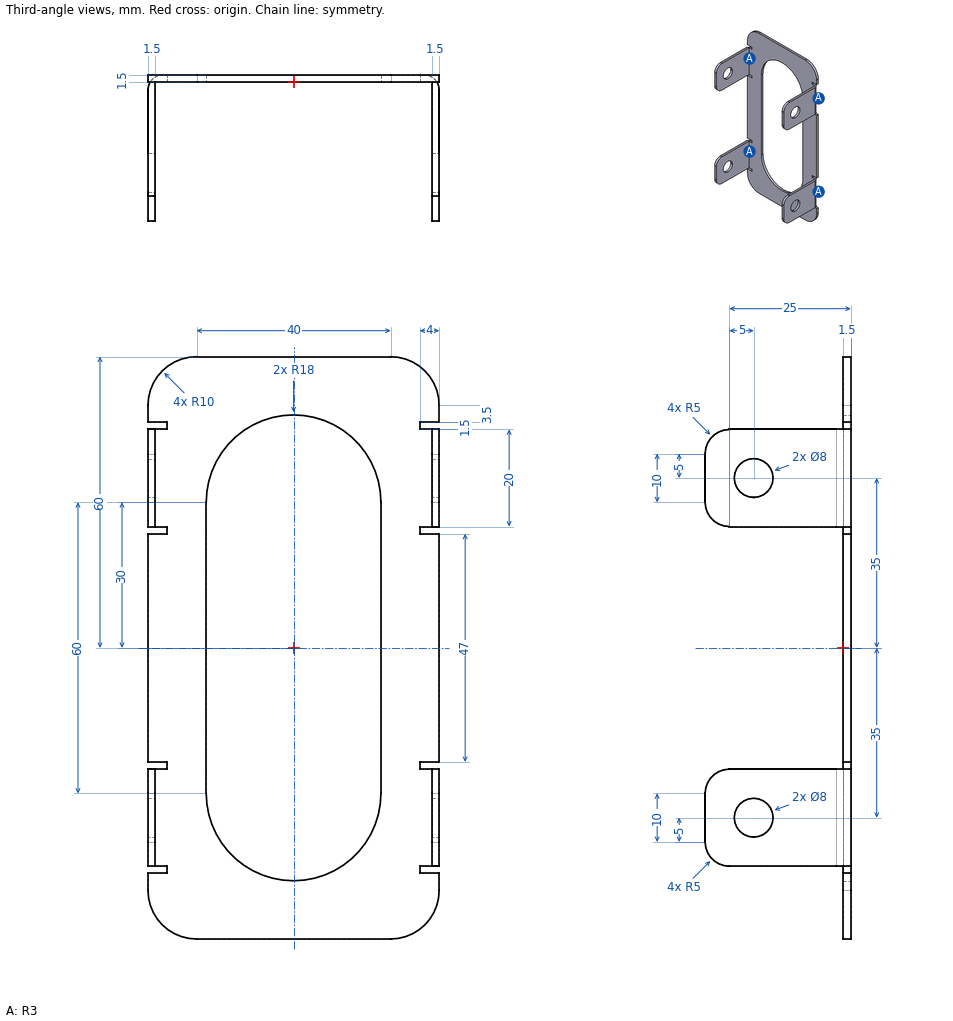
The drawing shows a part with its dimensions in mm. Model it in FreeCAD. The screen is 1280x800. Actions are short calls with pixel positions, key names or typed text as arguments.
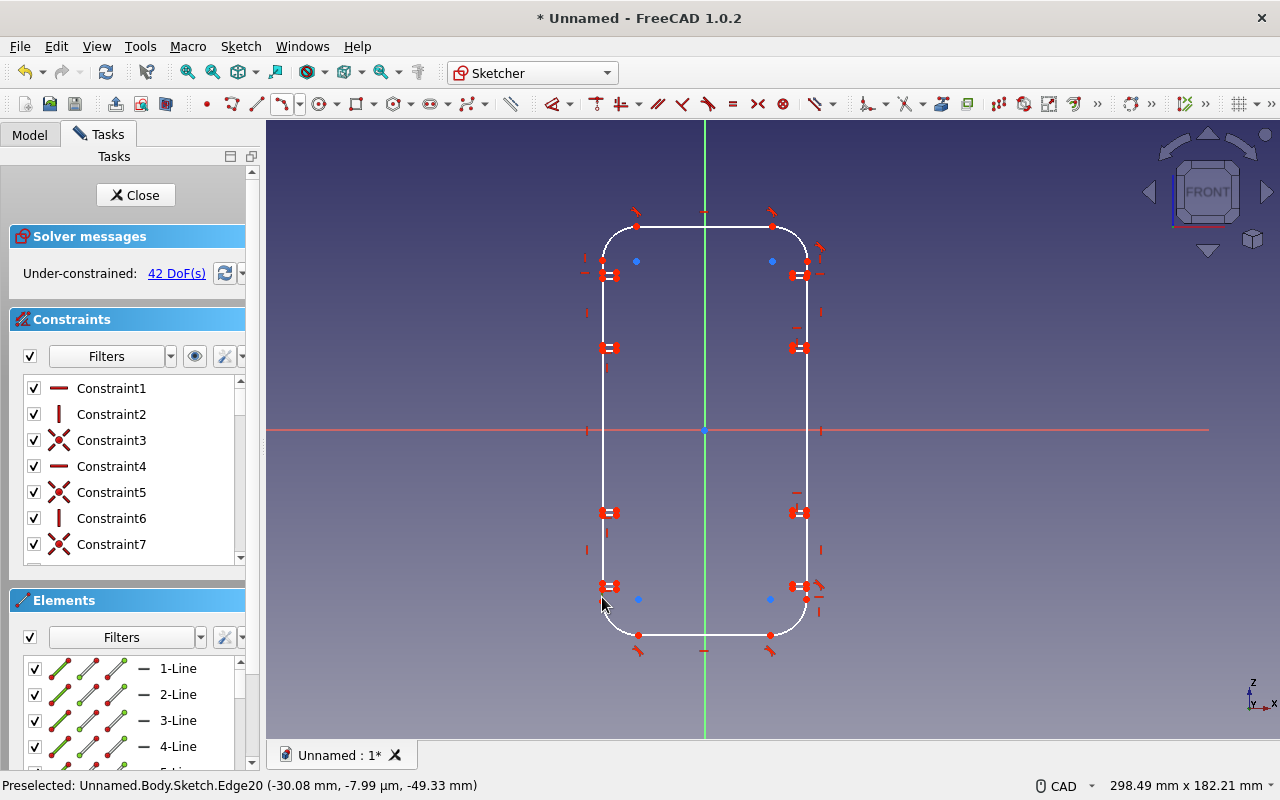
click(607, 617)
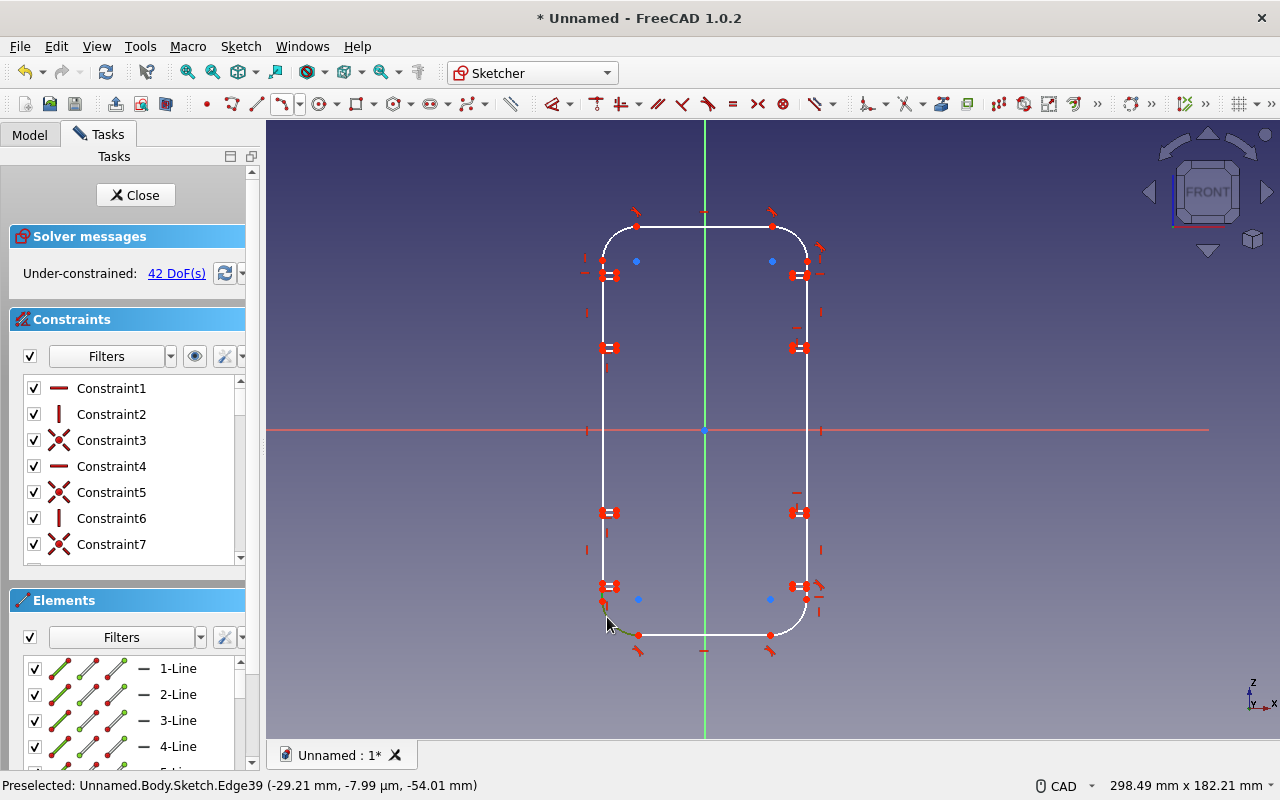
click(708, 104)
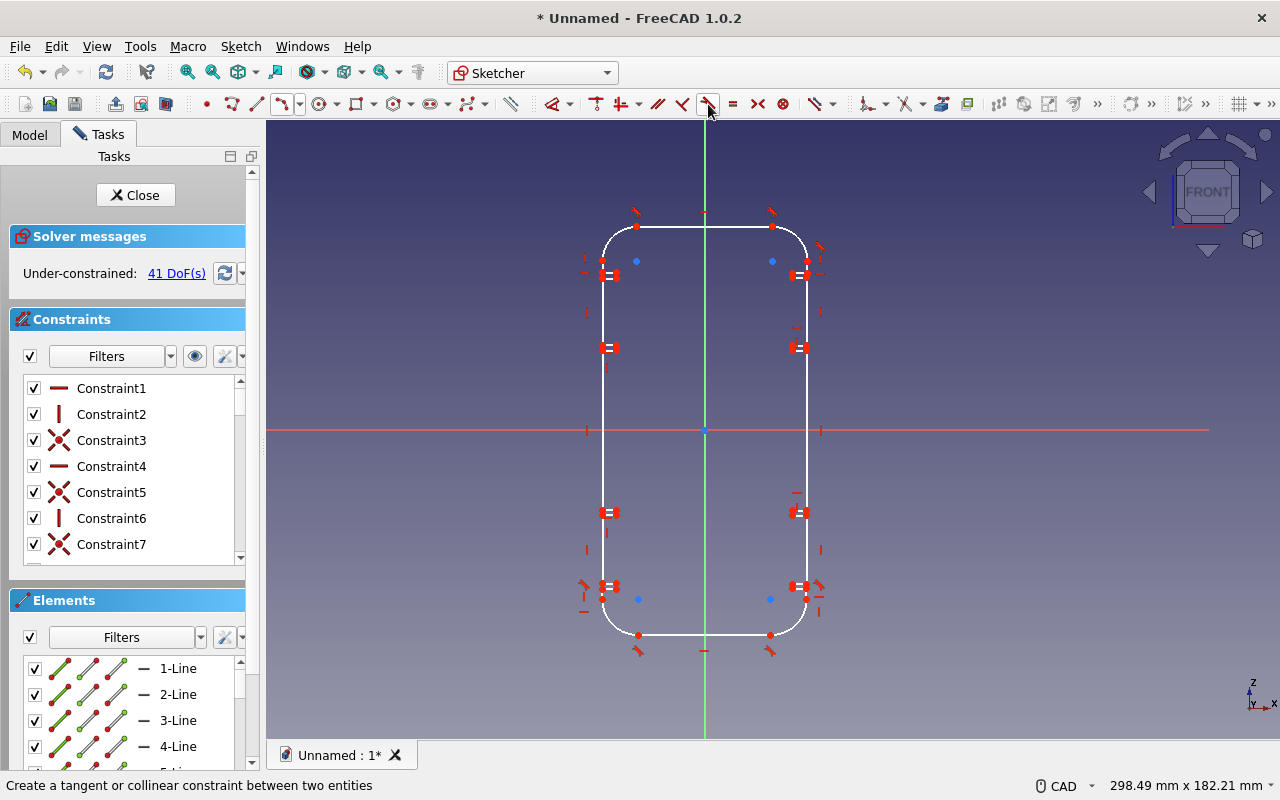
scroll(603, 267, up, 5)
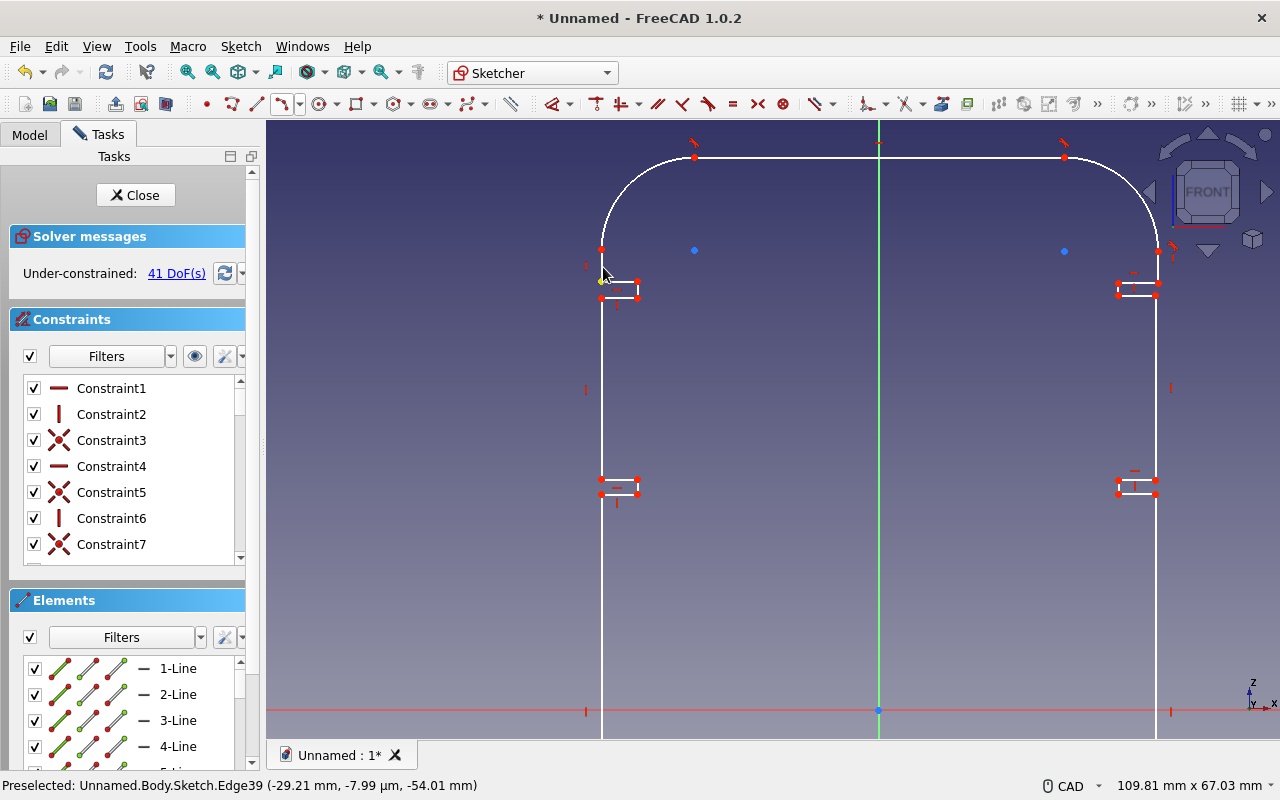
click(602, 266)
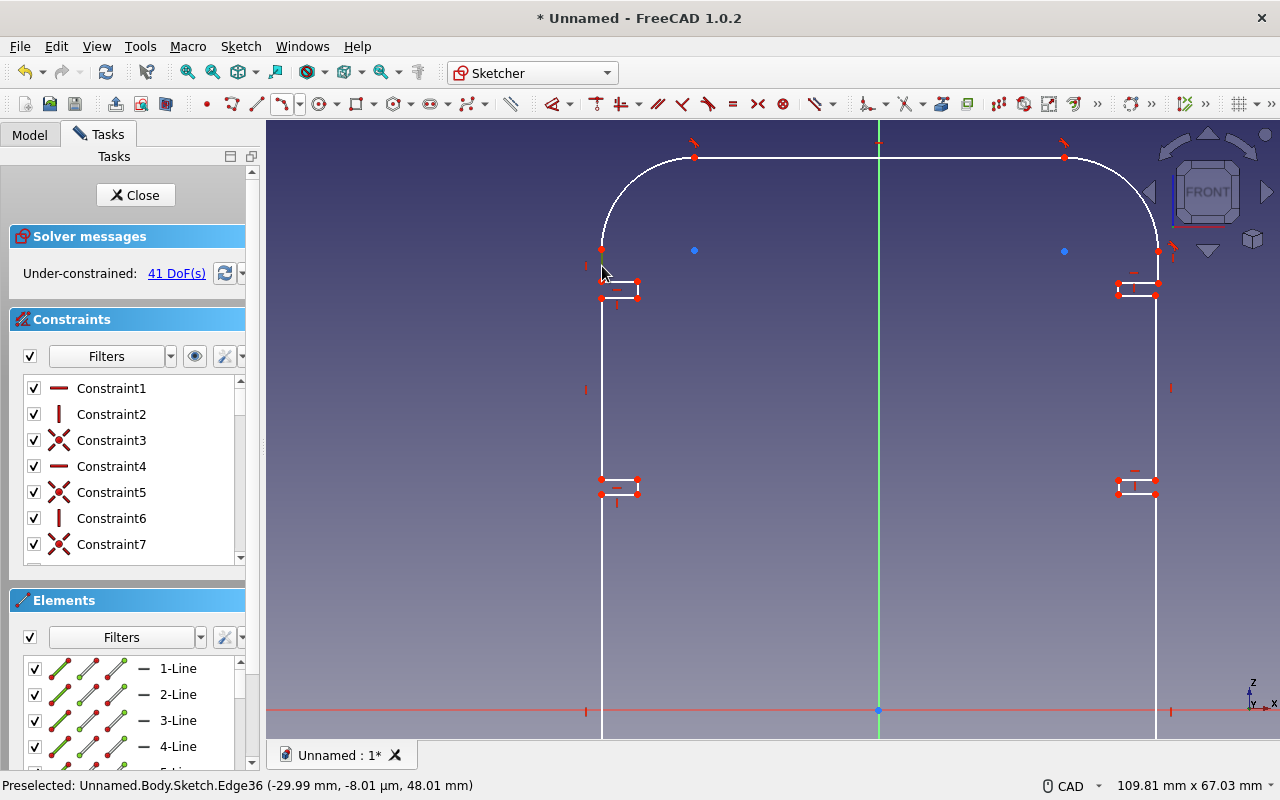
click(653, 168)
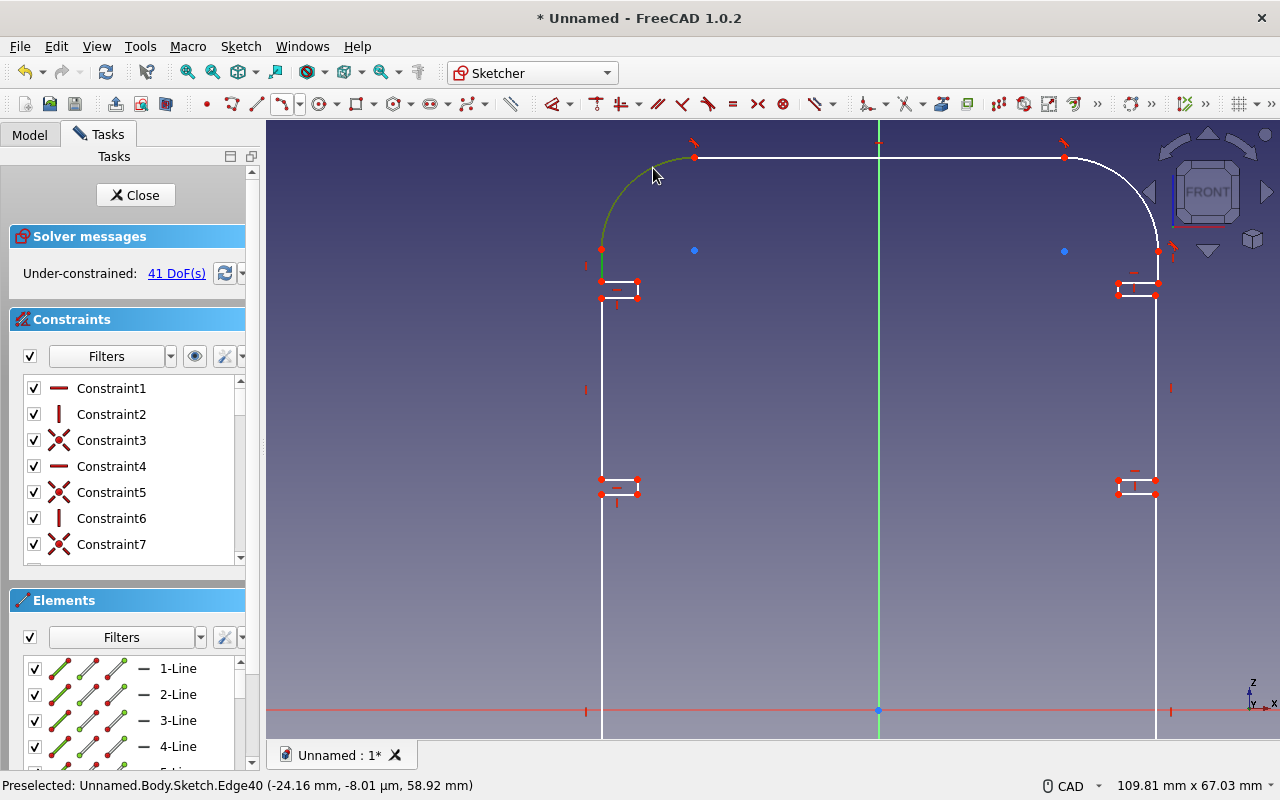
click(708, 104)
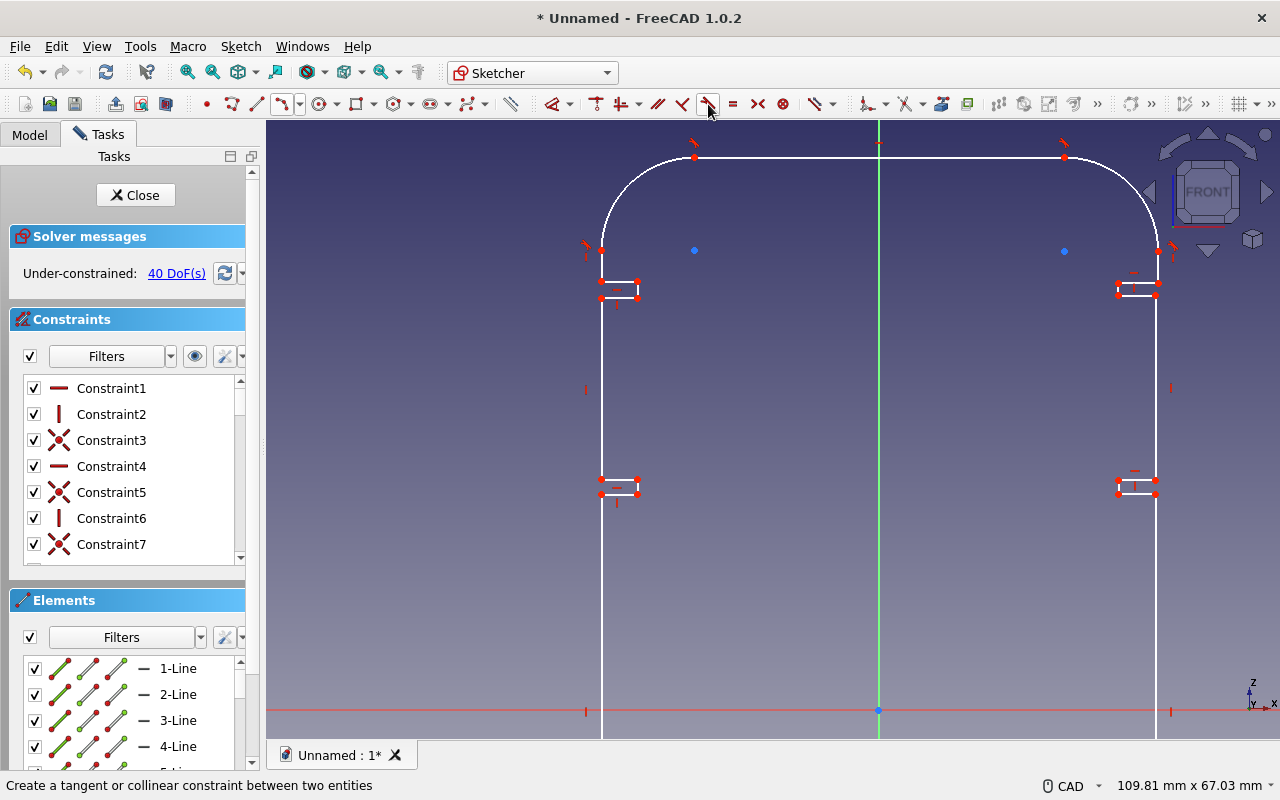
click(1107, 168)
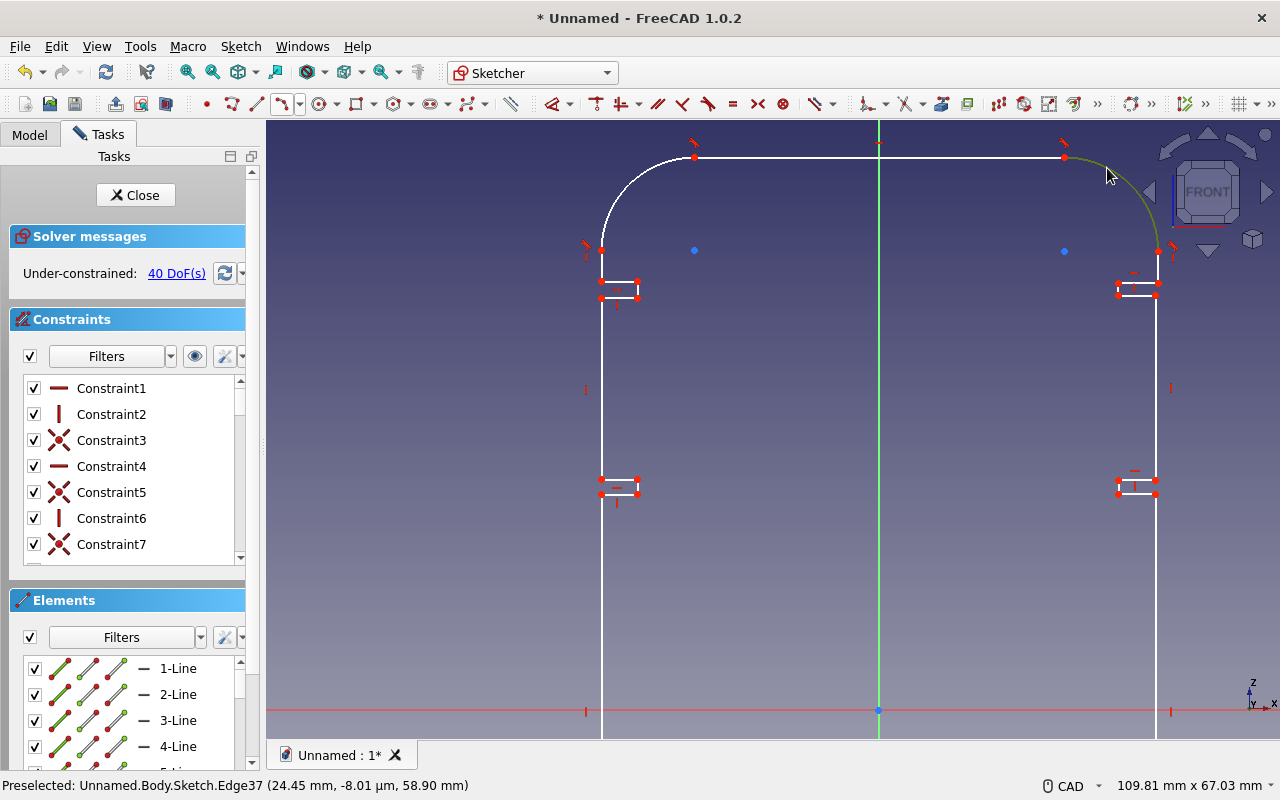
scroll(603, 266, down, 5)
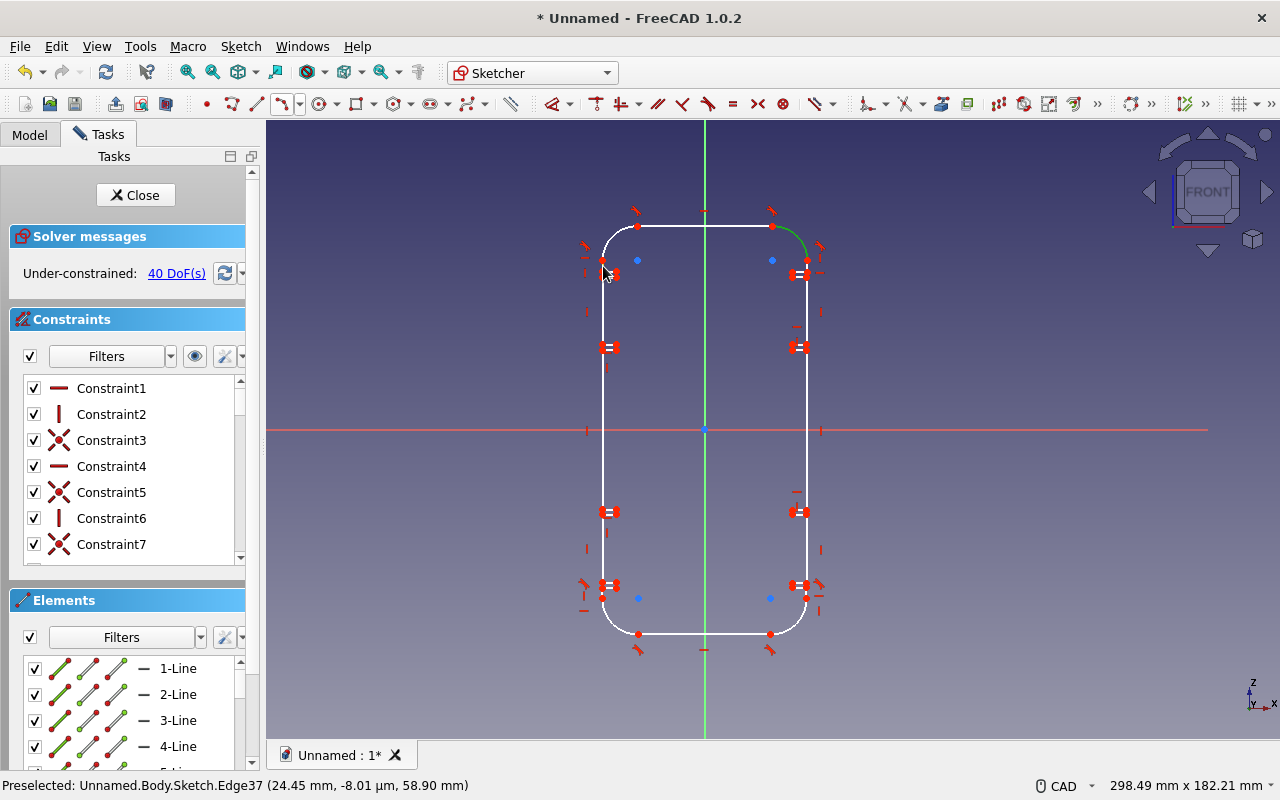
click(787, 631)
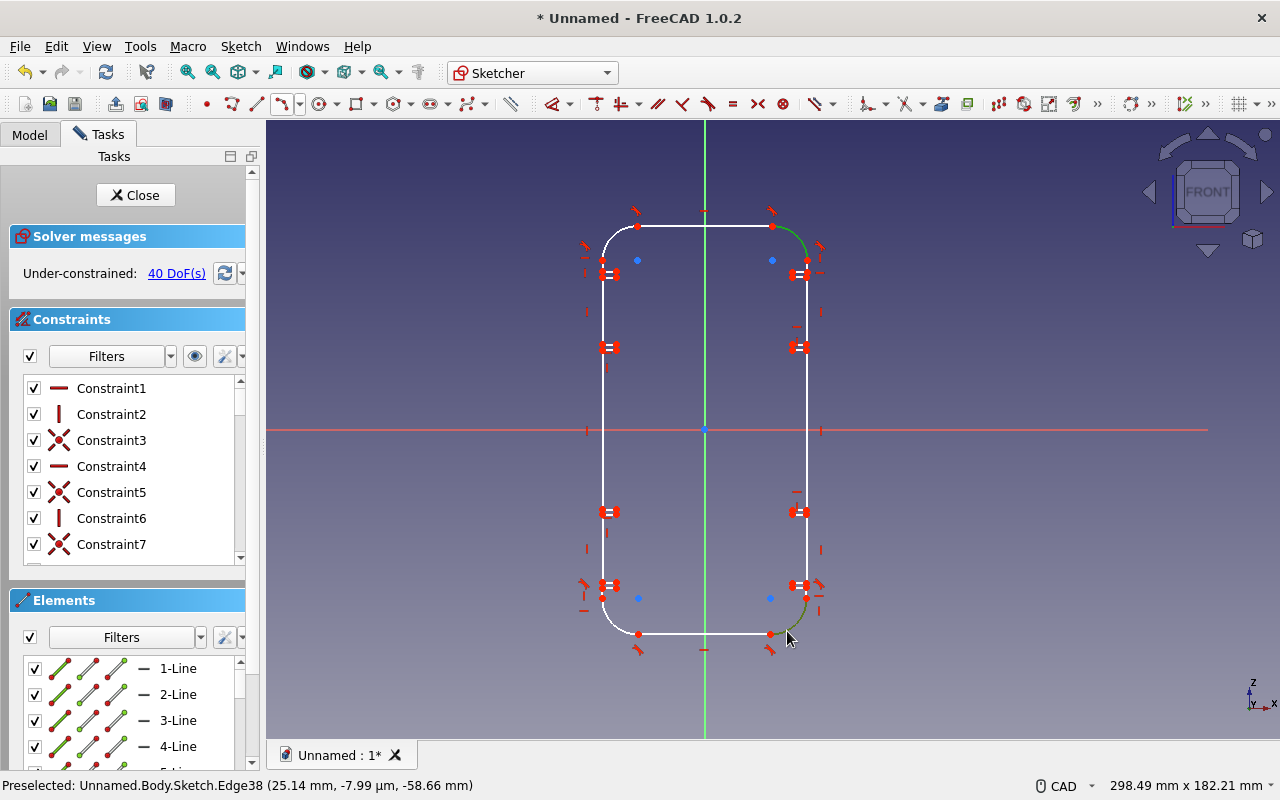
click(606, 615)